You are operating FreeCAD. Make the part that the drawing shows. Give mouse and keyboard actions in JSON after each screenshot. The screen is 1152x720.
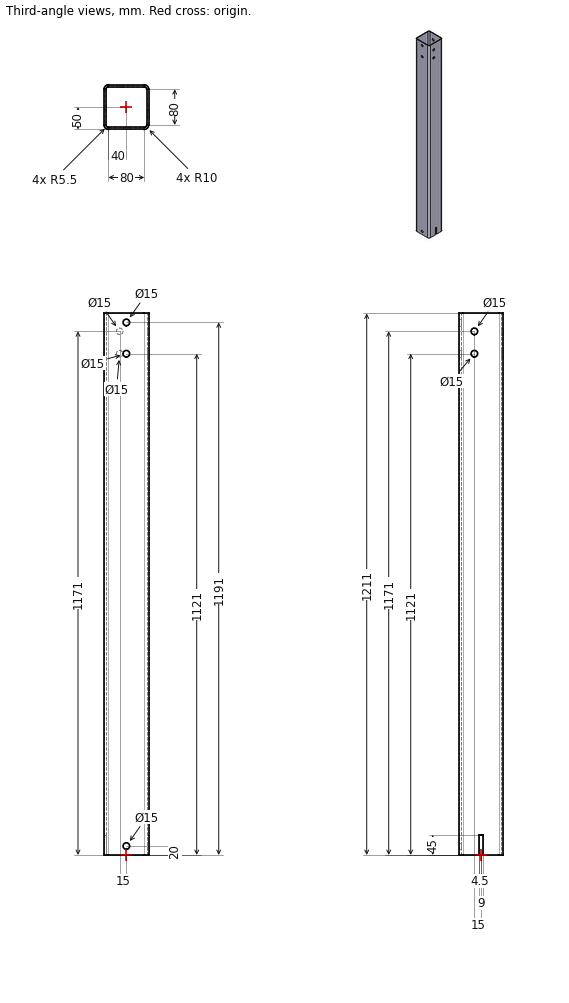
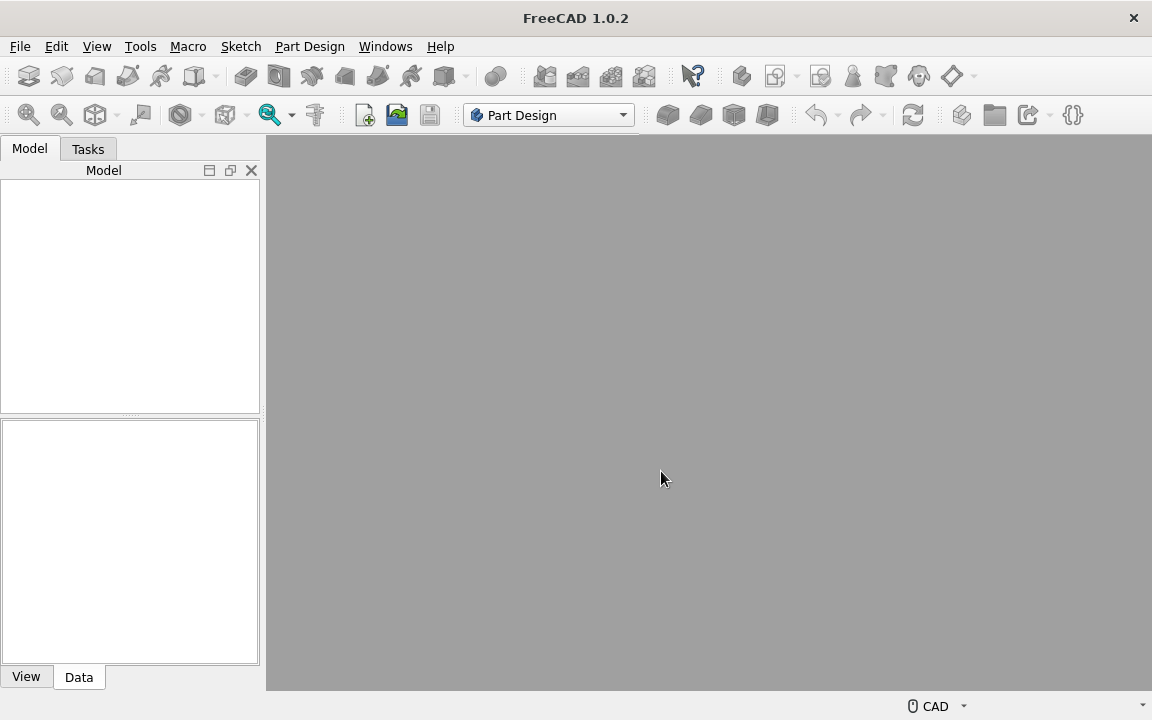
{"action": "key", "text": "ctrl+n"}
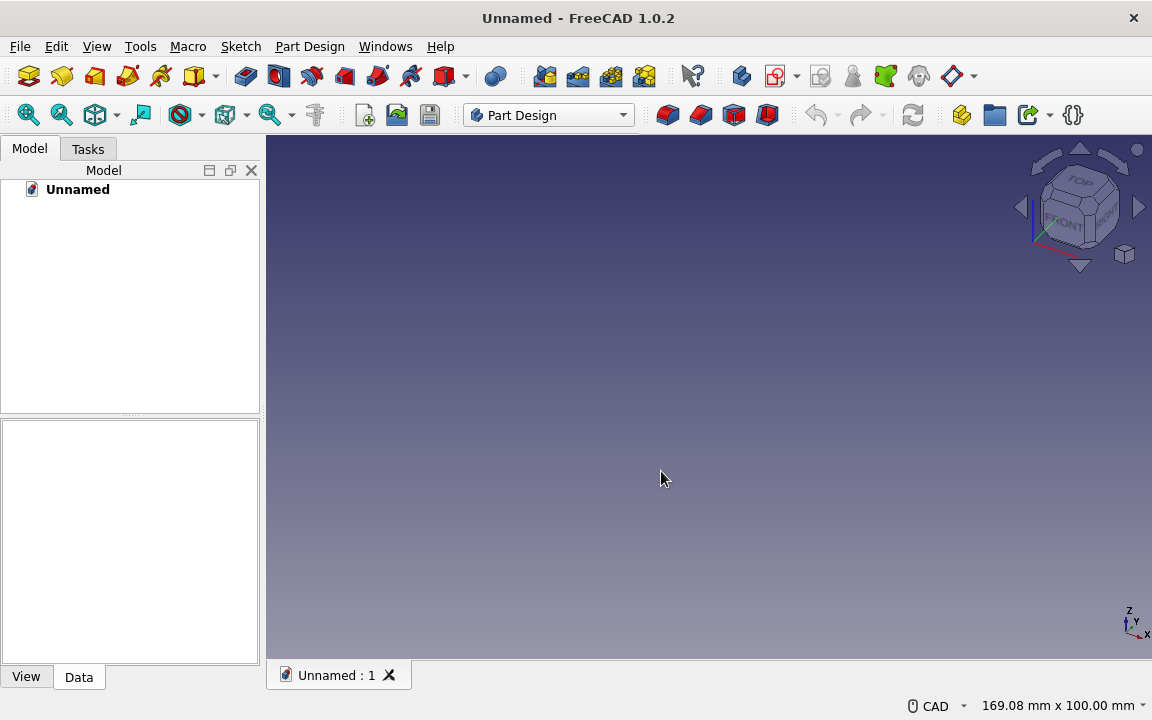
{"action": "left_click", "coordinate": [774, 76]}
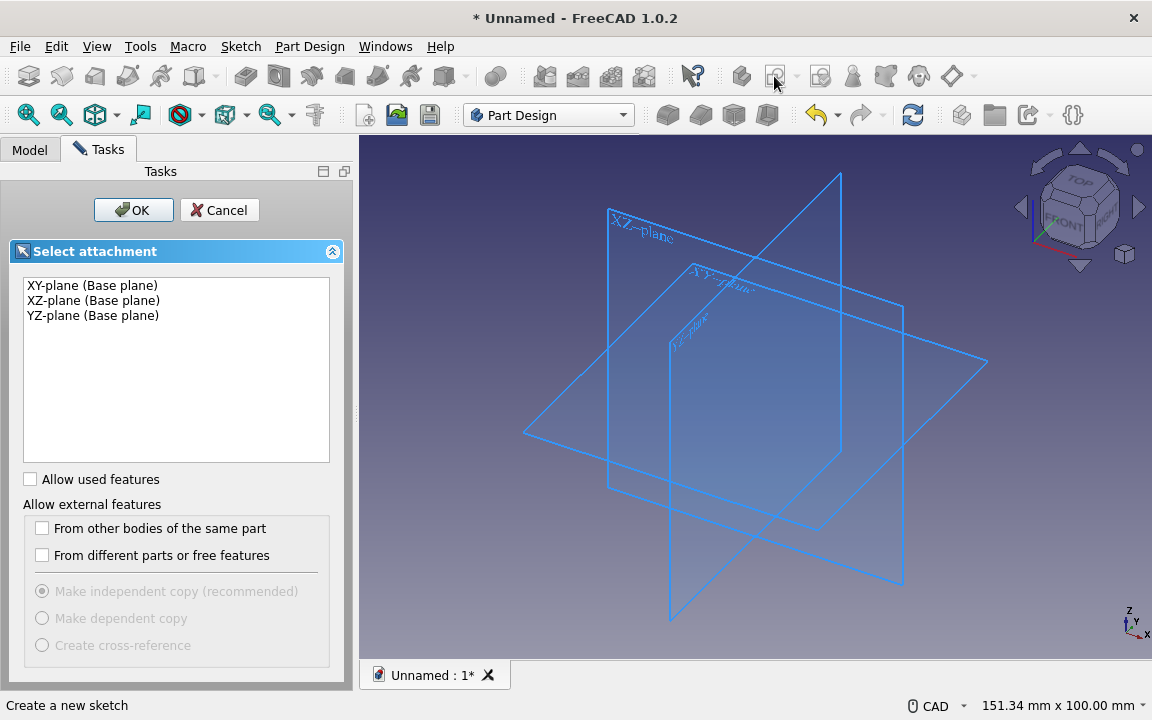
{"action": "left_click", "coordinate": [84, 286]}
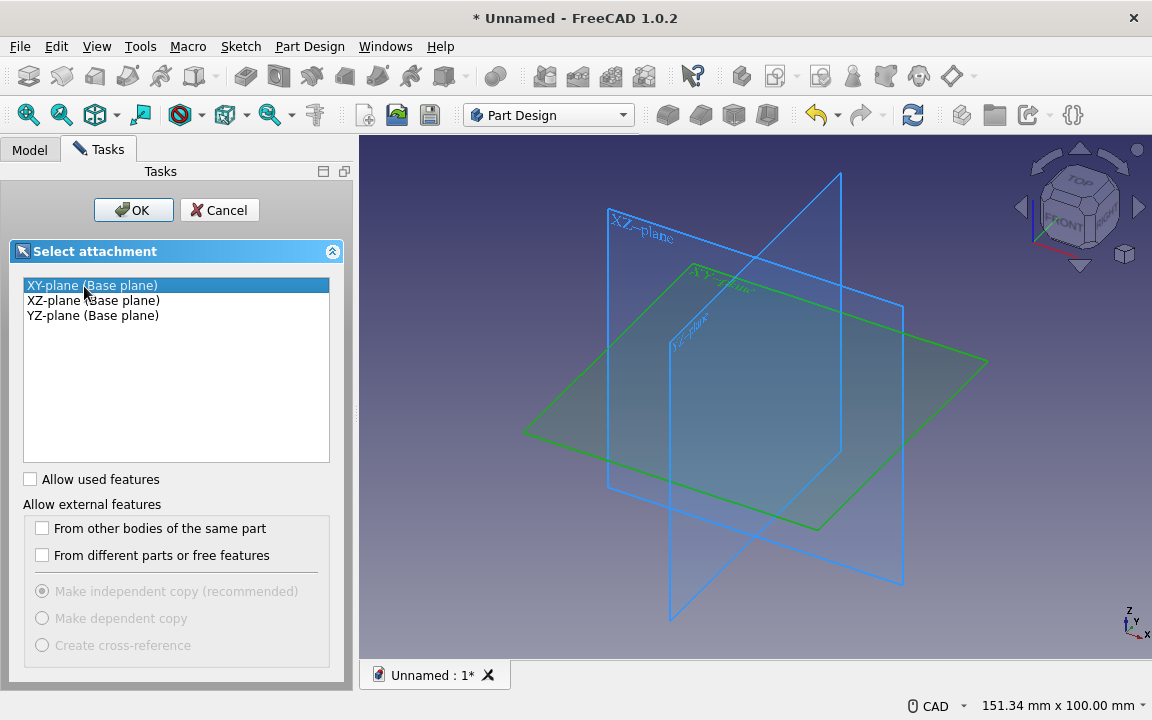
{"action": "left_click", "coordinate": [134, 210]}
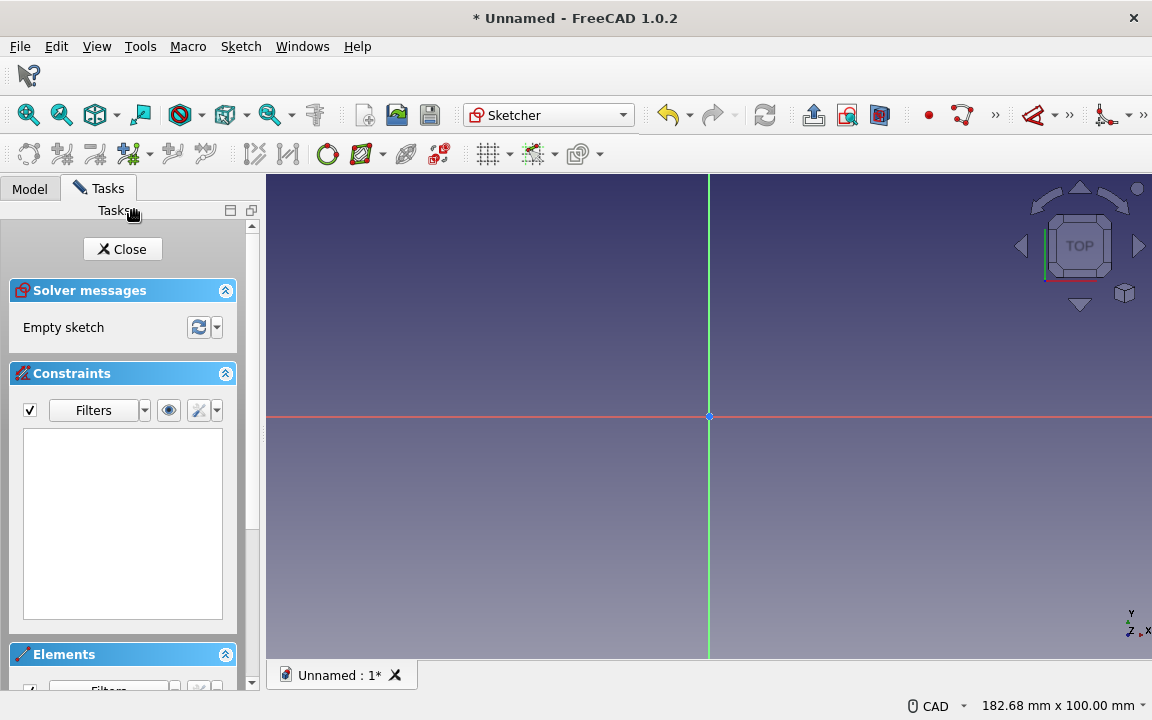
{"action": "scroll", "coordinate": [501, 416], "scroll_direction": "down", "scroll_amount": 2}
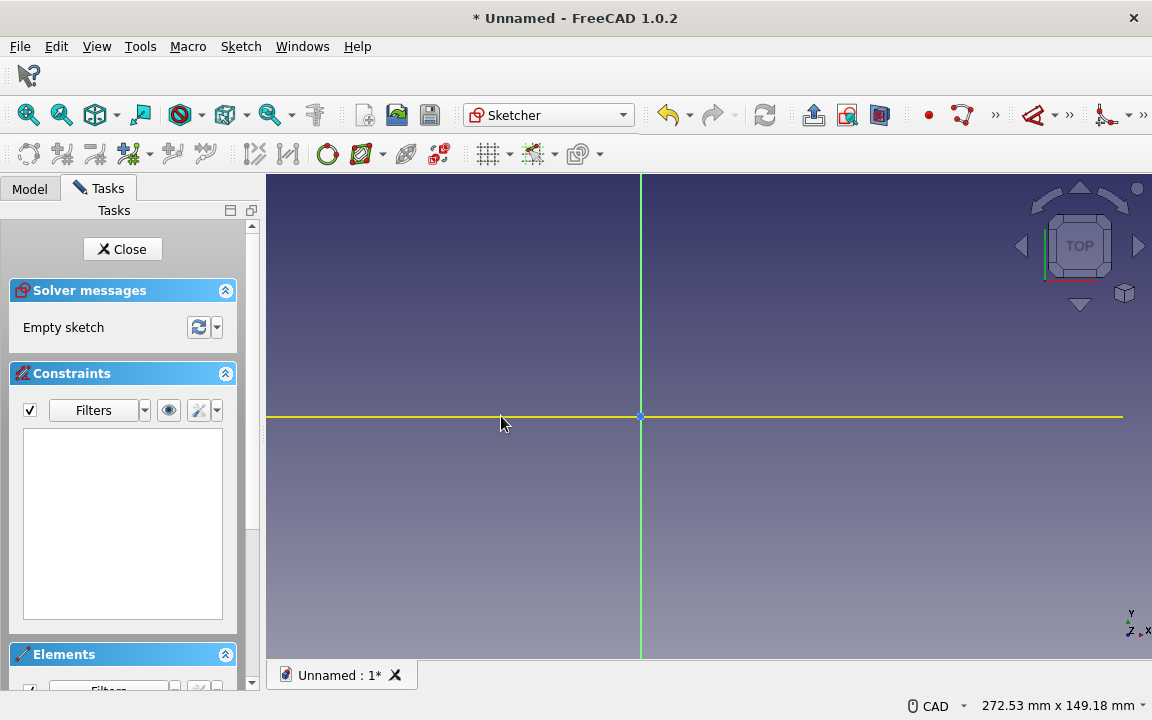
{"action": "key", "text": "g l"}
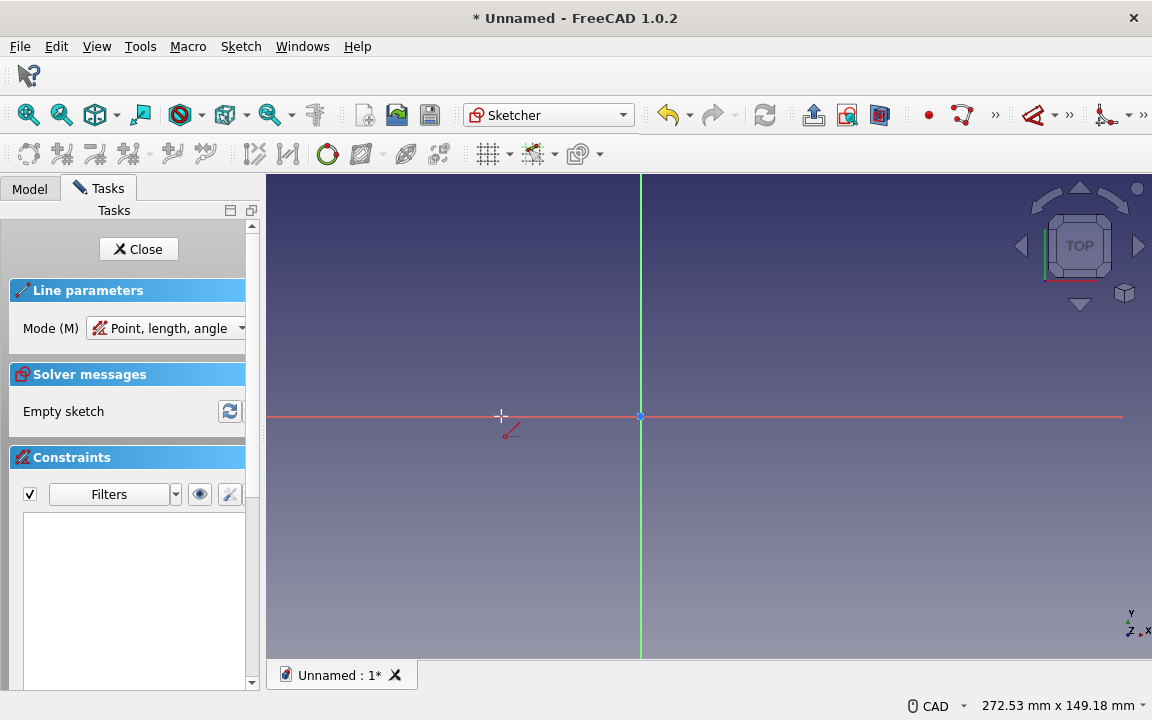
{"action": "left_click", "coordinate": [510, 579]}
{"action": "left_click", "coordinate": [771, 579]}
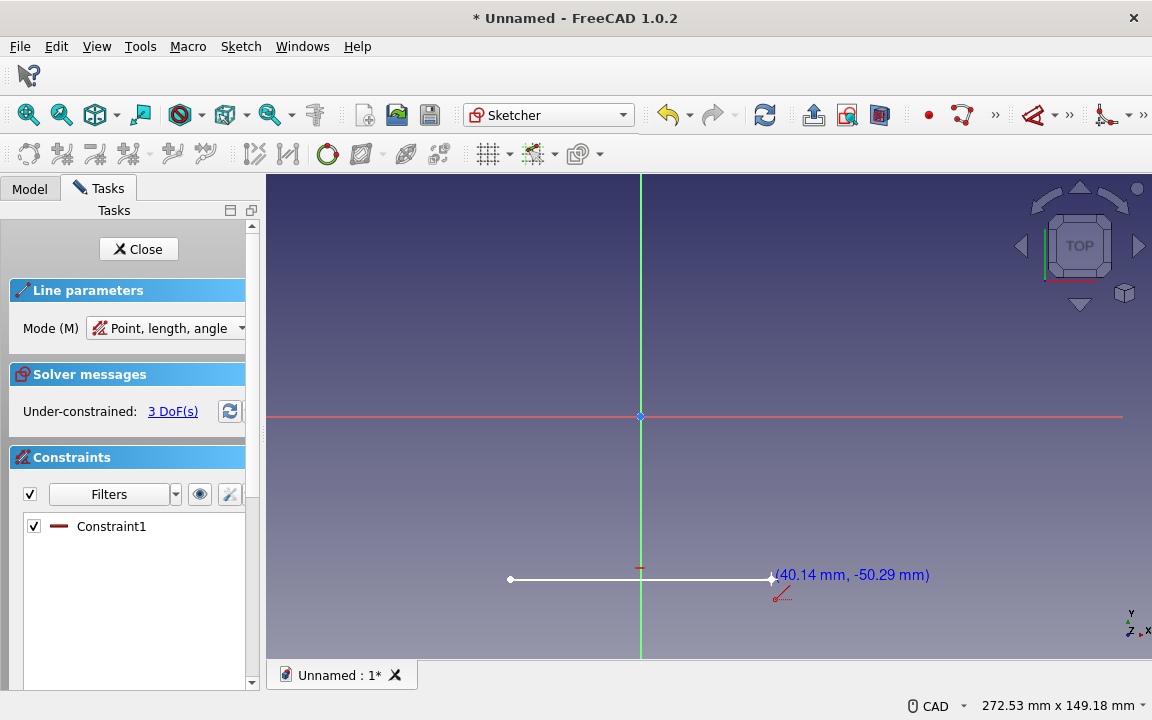
{"action": "left_click", "coordinate": [803, 547]}
{"action": "left_click", "coordinate": [803, 286]}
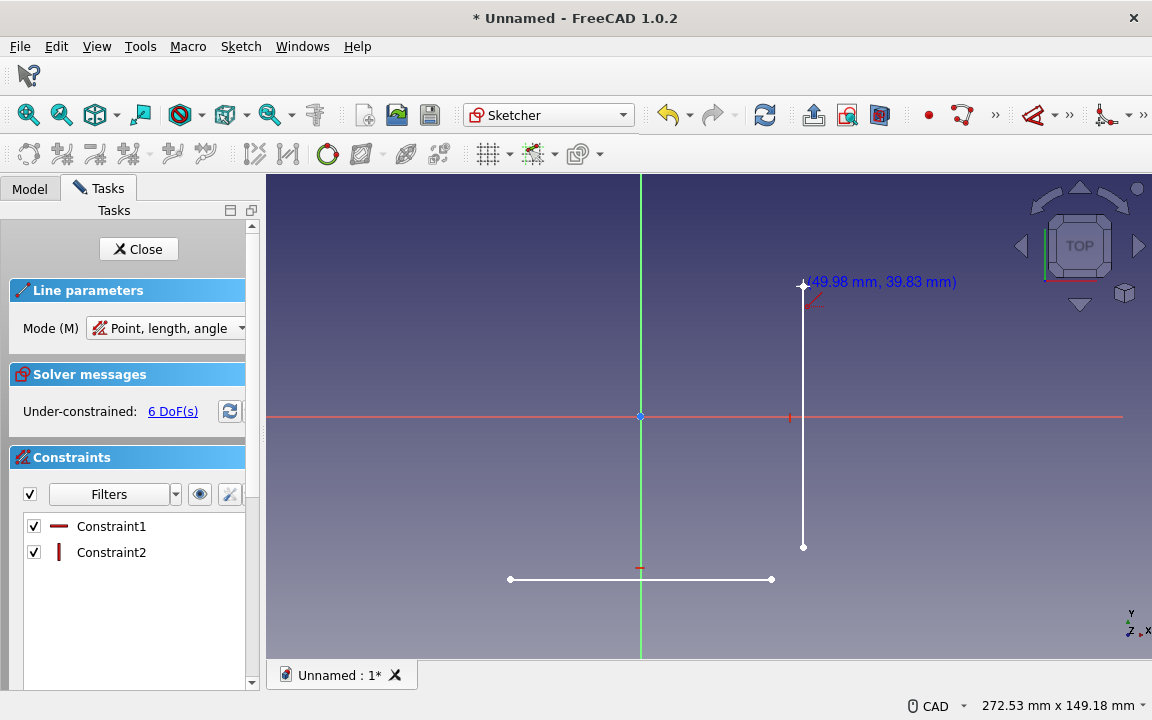
{"action": "left_click", "coordinate": [771, 254]}
{"action": "left_click", "coordinate": [510, 254]}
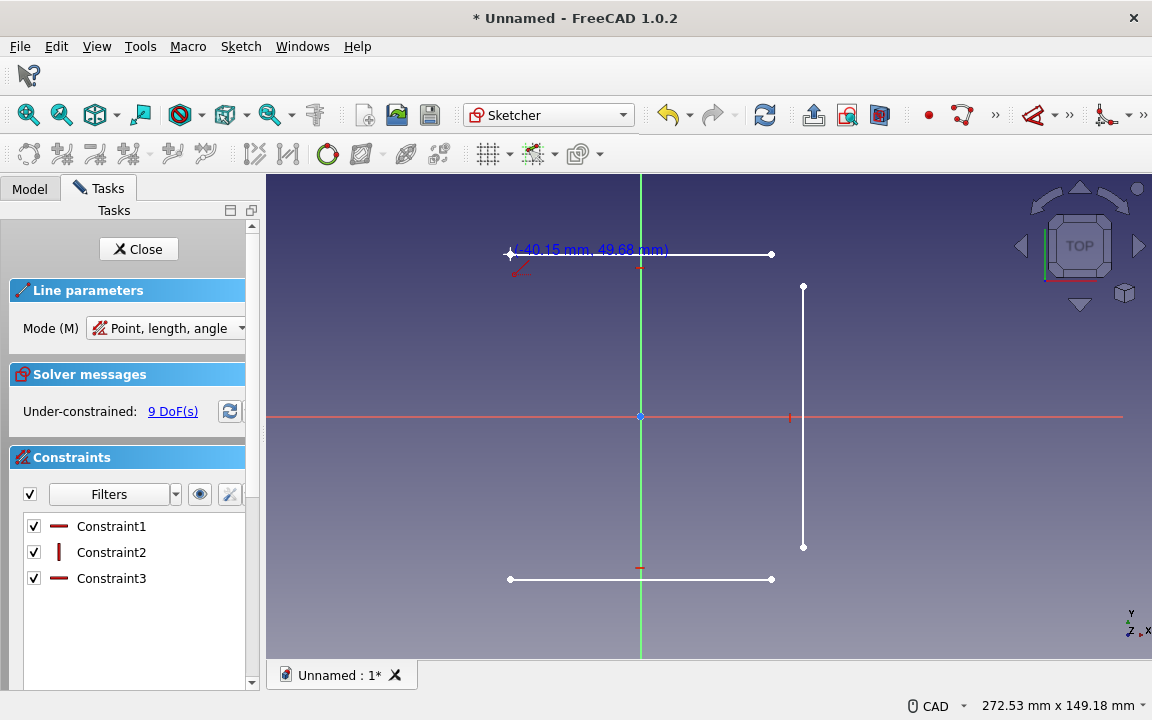
{"action": "left_click", "coordinate": [478, 286]}
{"action": "left_click", "coordinate": [478, 547]}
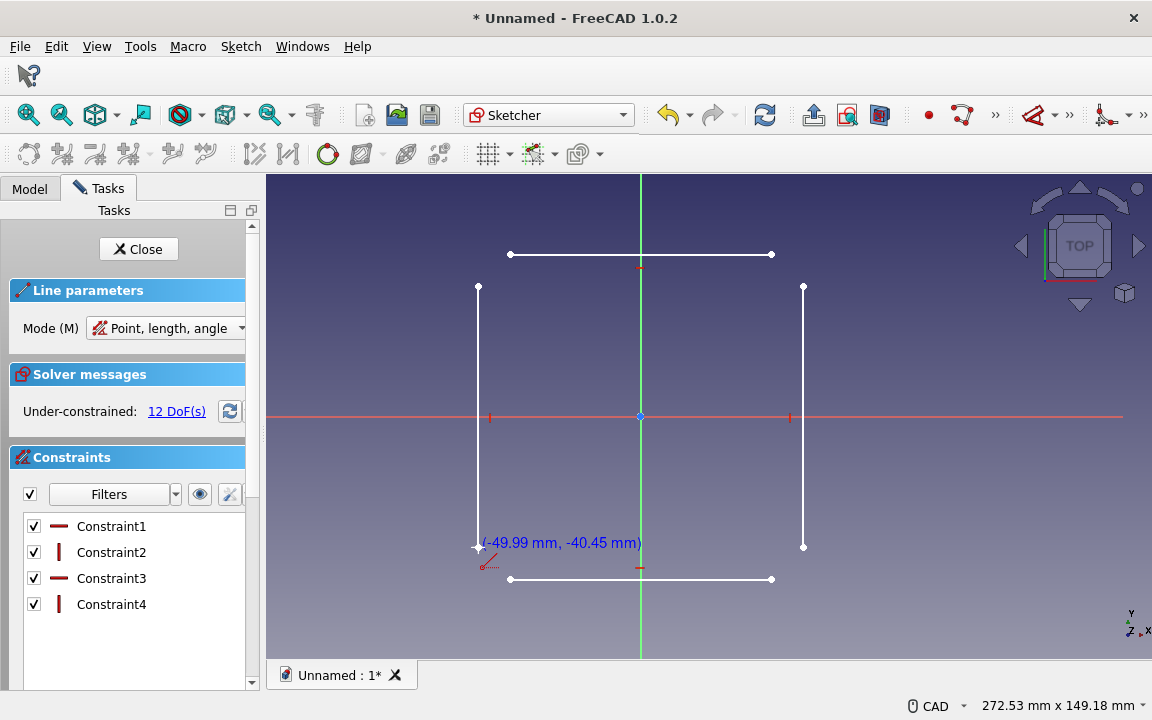
{"action": "key", "text": "g 3 a"}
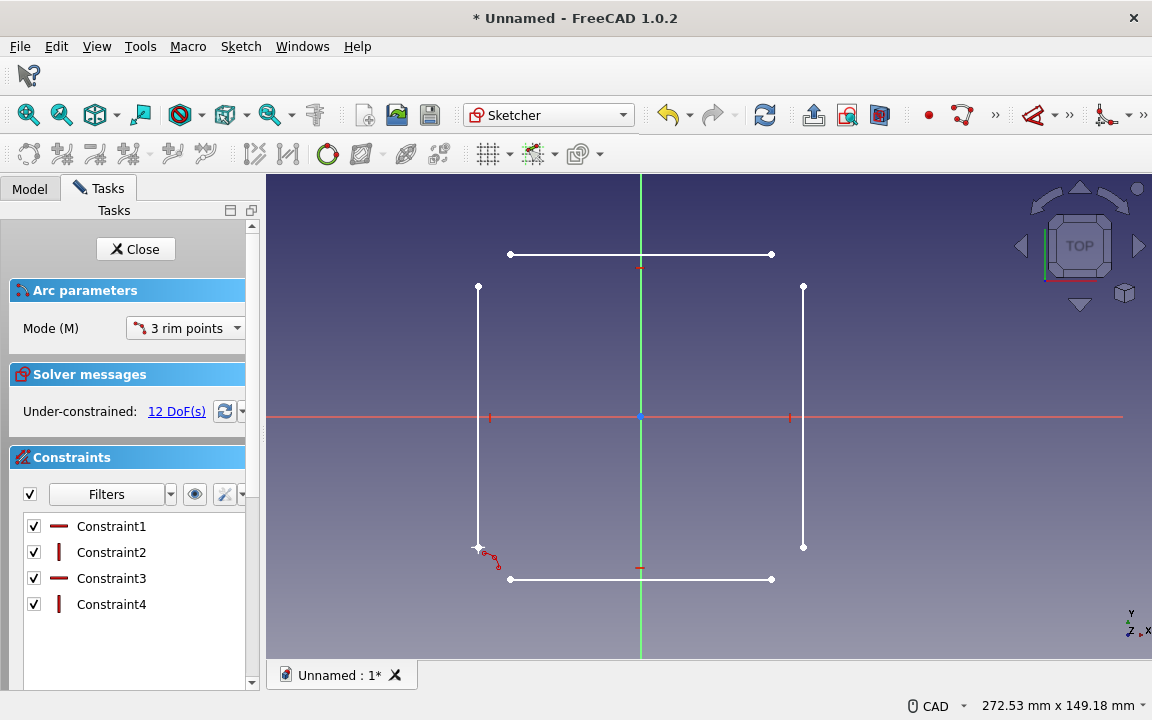
{"action": "left_click", "coordinate": [771, 580]}
{"action": "left_click", "coordinate": [803, 548]}